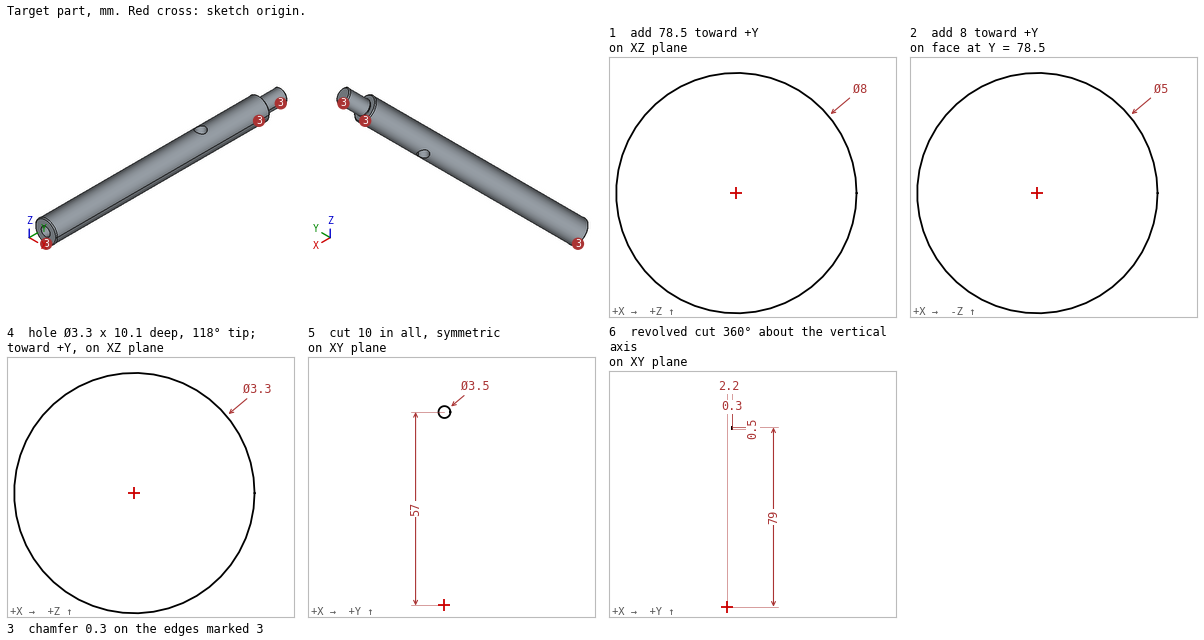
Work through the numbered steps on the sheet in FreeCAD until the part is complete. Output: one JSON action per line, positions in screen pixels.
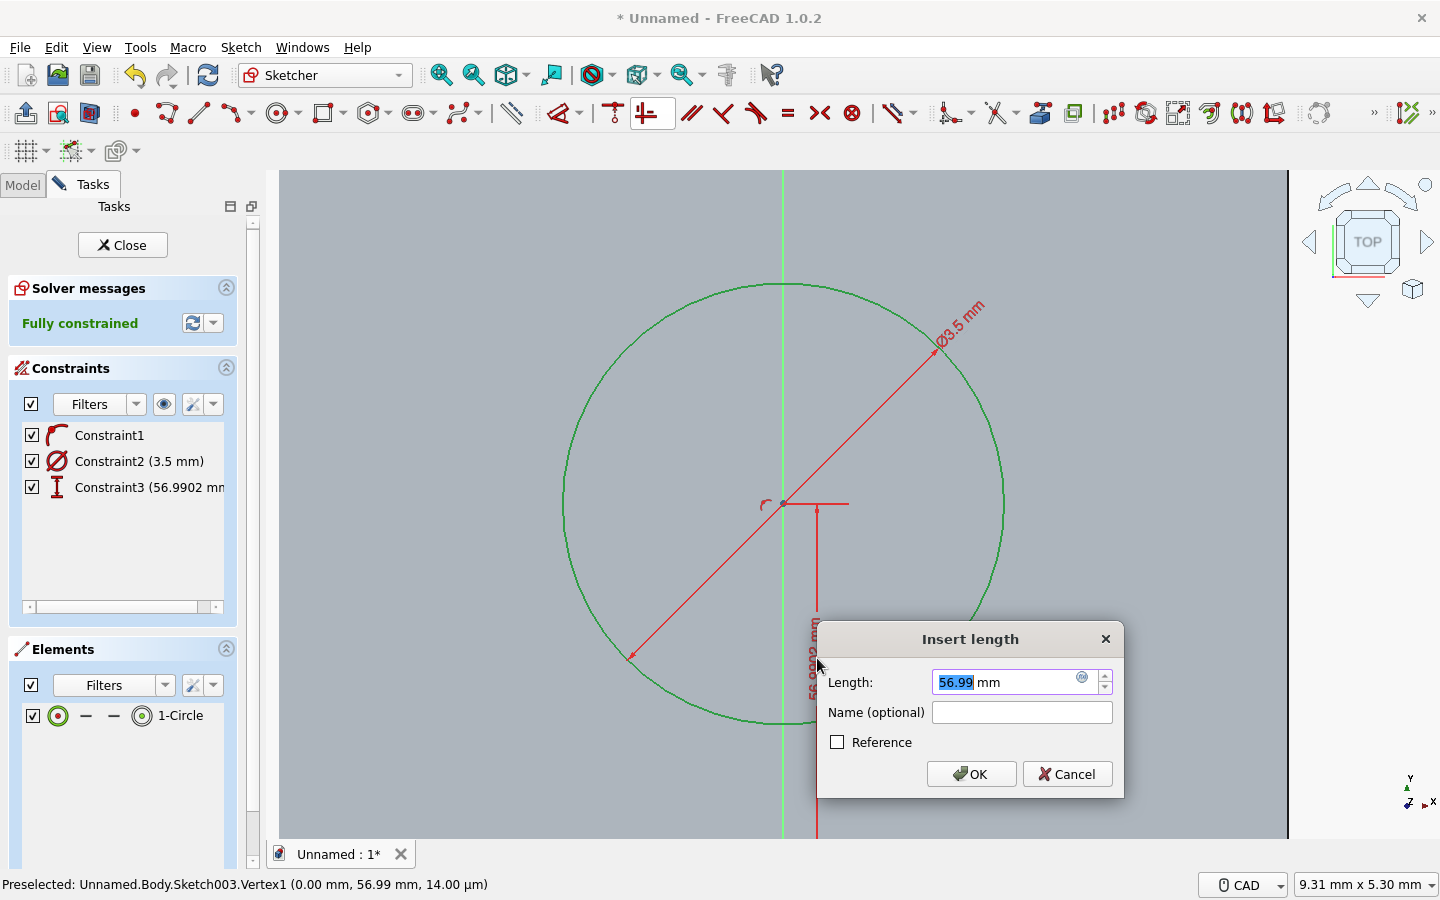
{"action": "type", "text": "57"}
{"action": "key", "text": "Return"}
{"action": "key", "text": "Escape"}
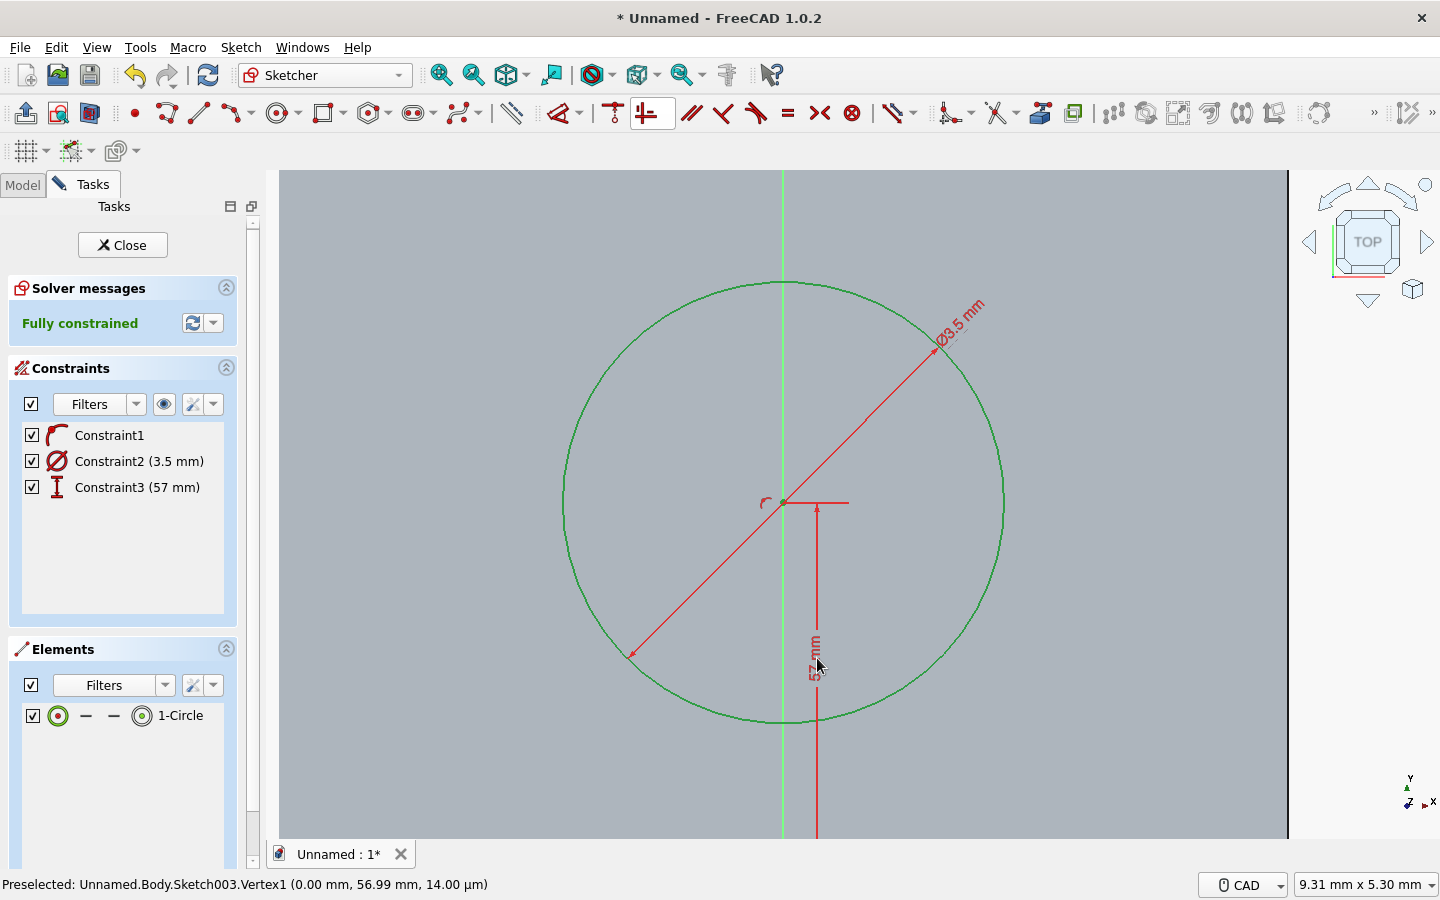
{"action": "left_click", "coordinate": [123, 245]}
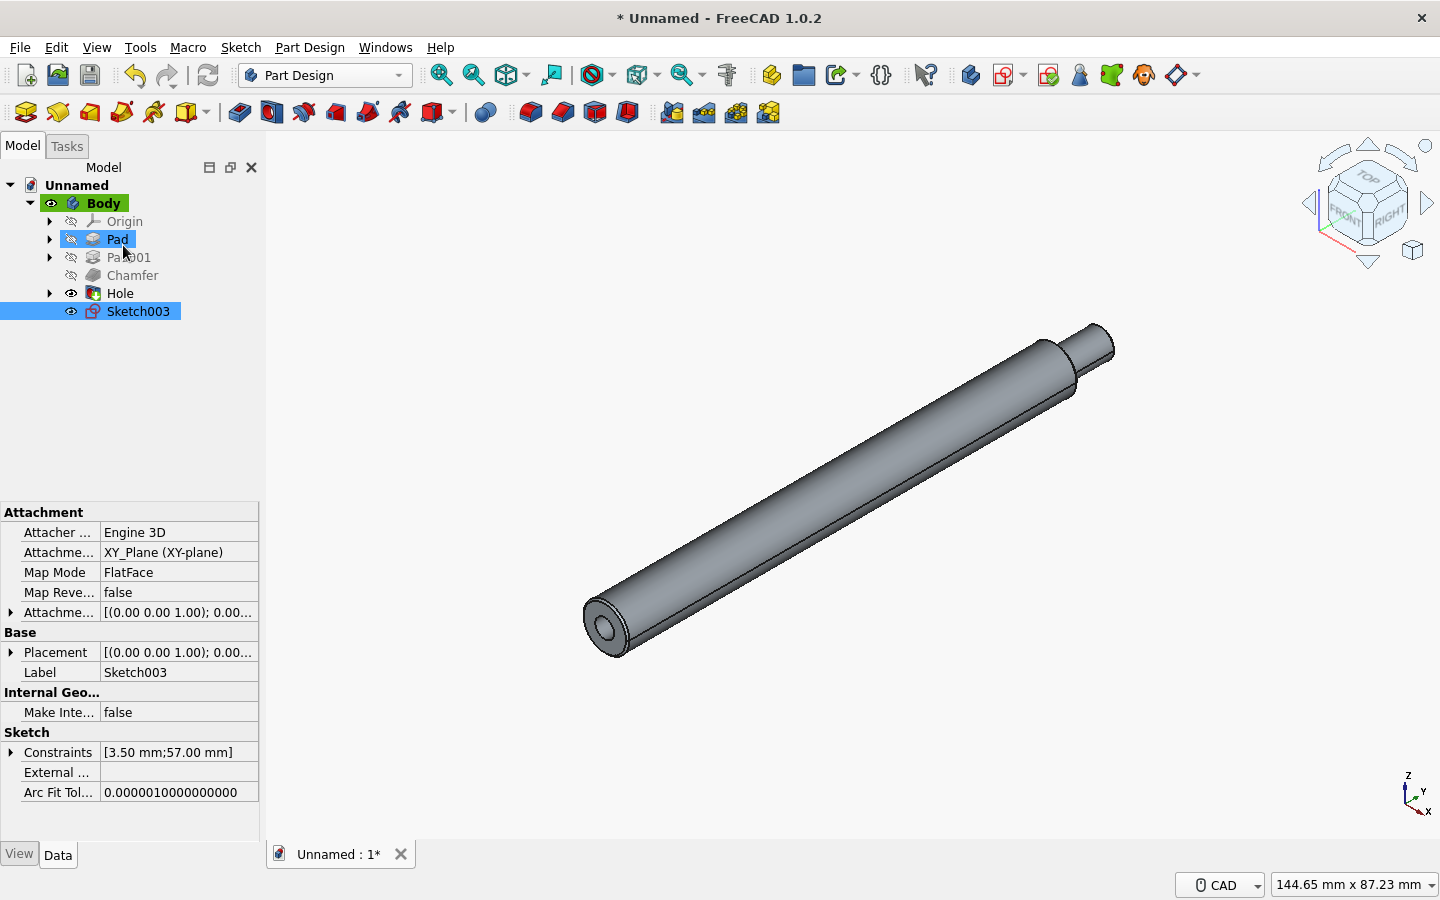
{"action": "left_click", "coordinate": [240, 112]}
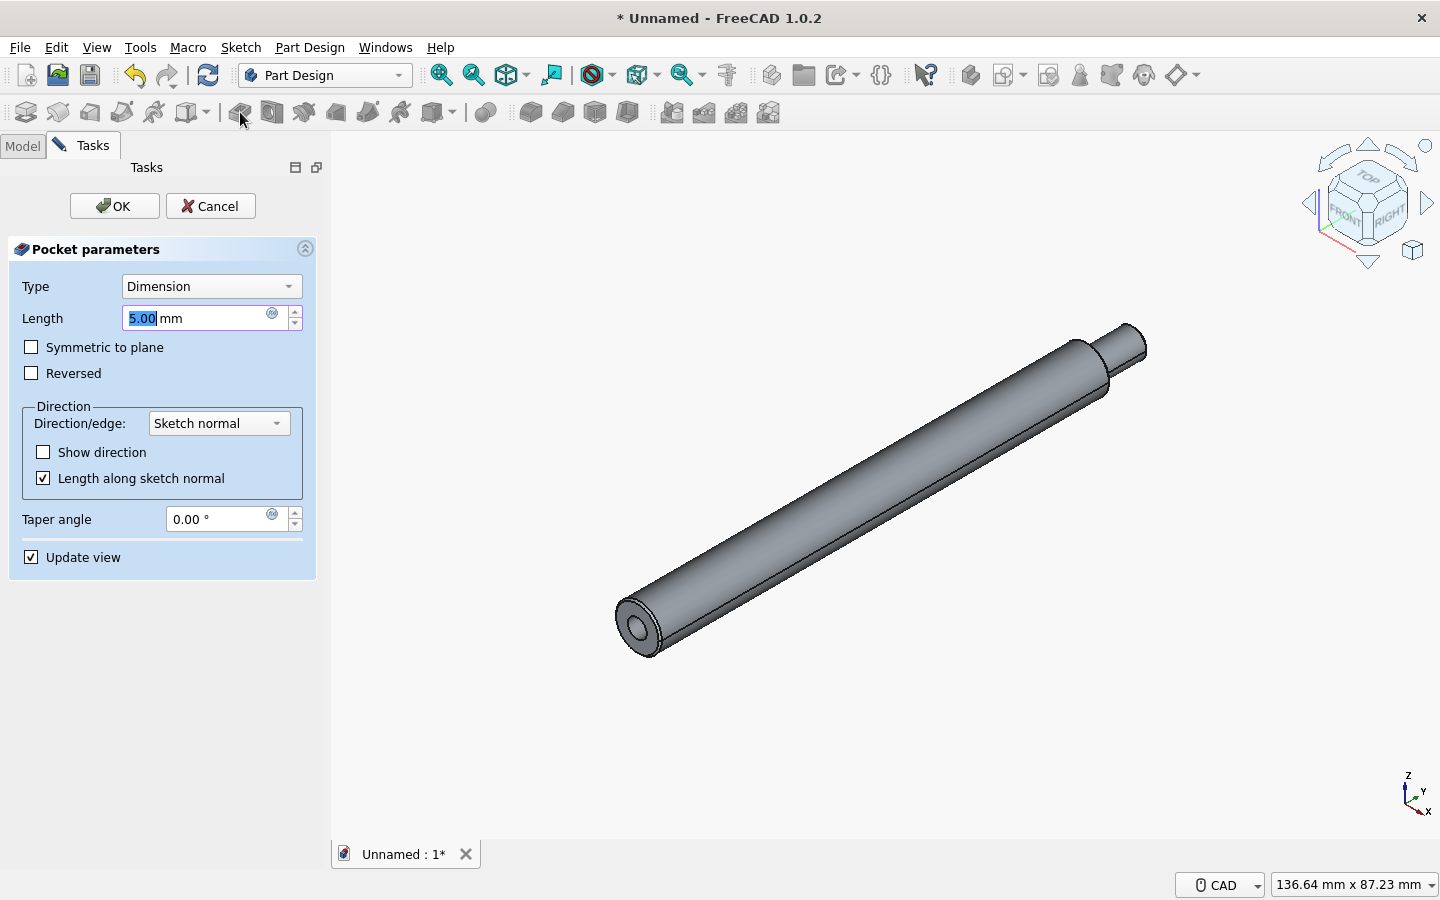
{"action": "type", "text": "10"}
{"action": "key", "text": "Tab"}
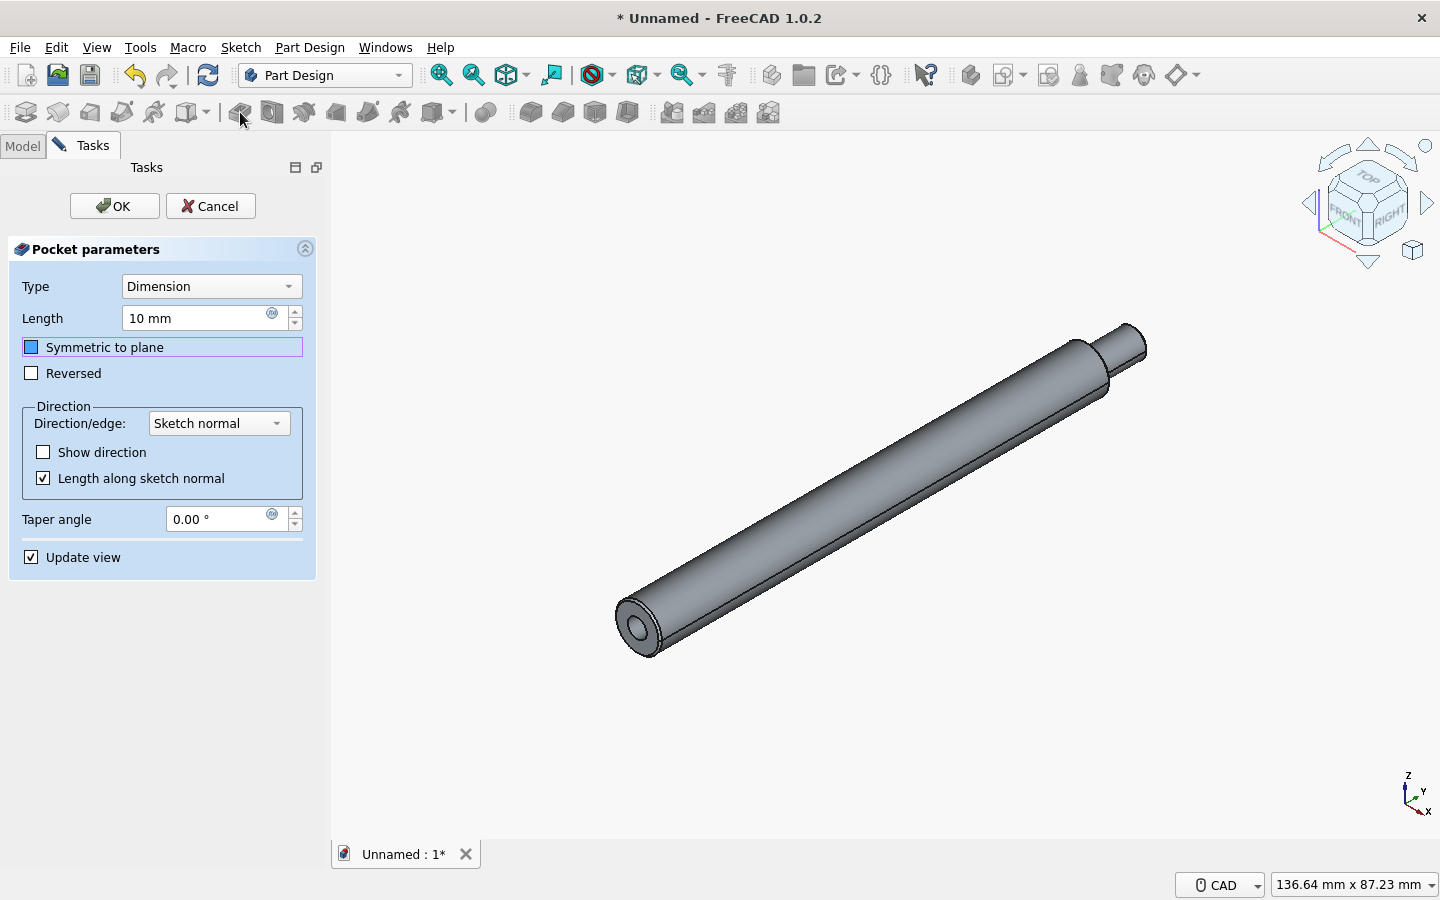
{"action": "left_click", "coordinate": [30, 347]}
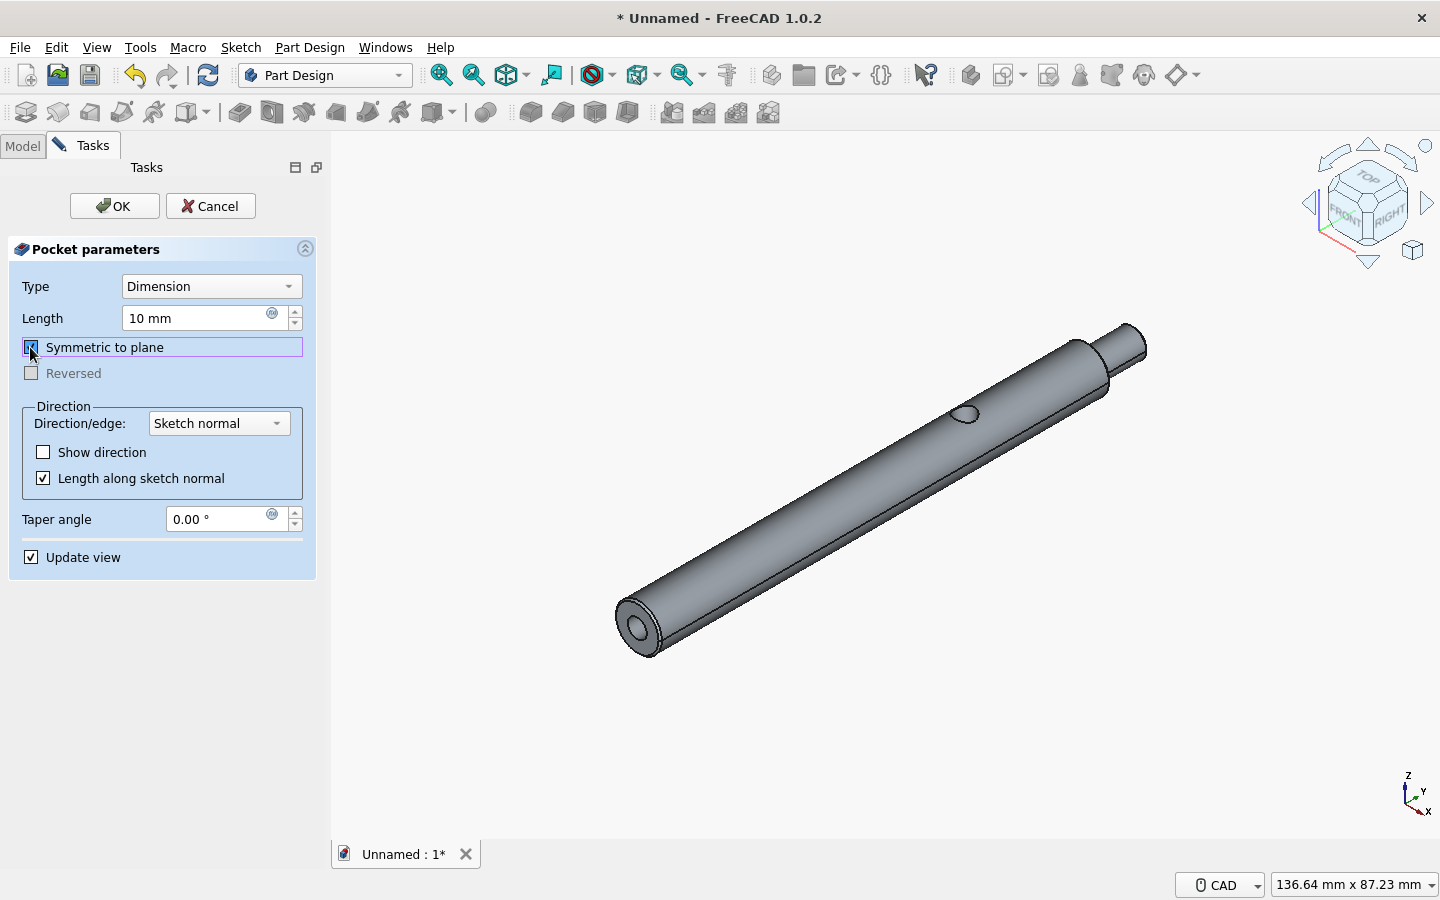
{"action": "left_click", "coordinate": [115, 206]}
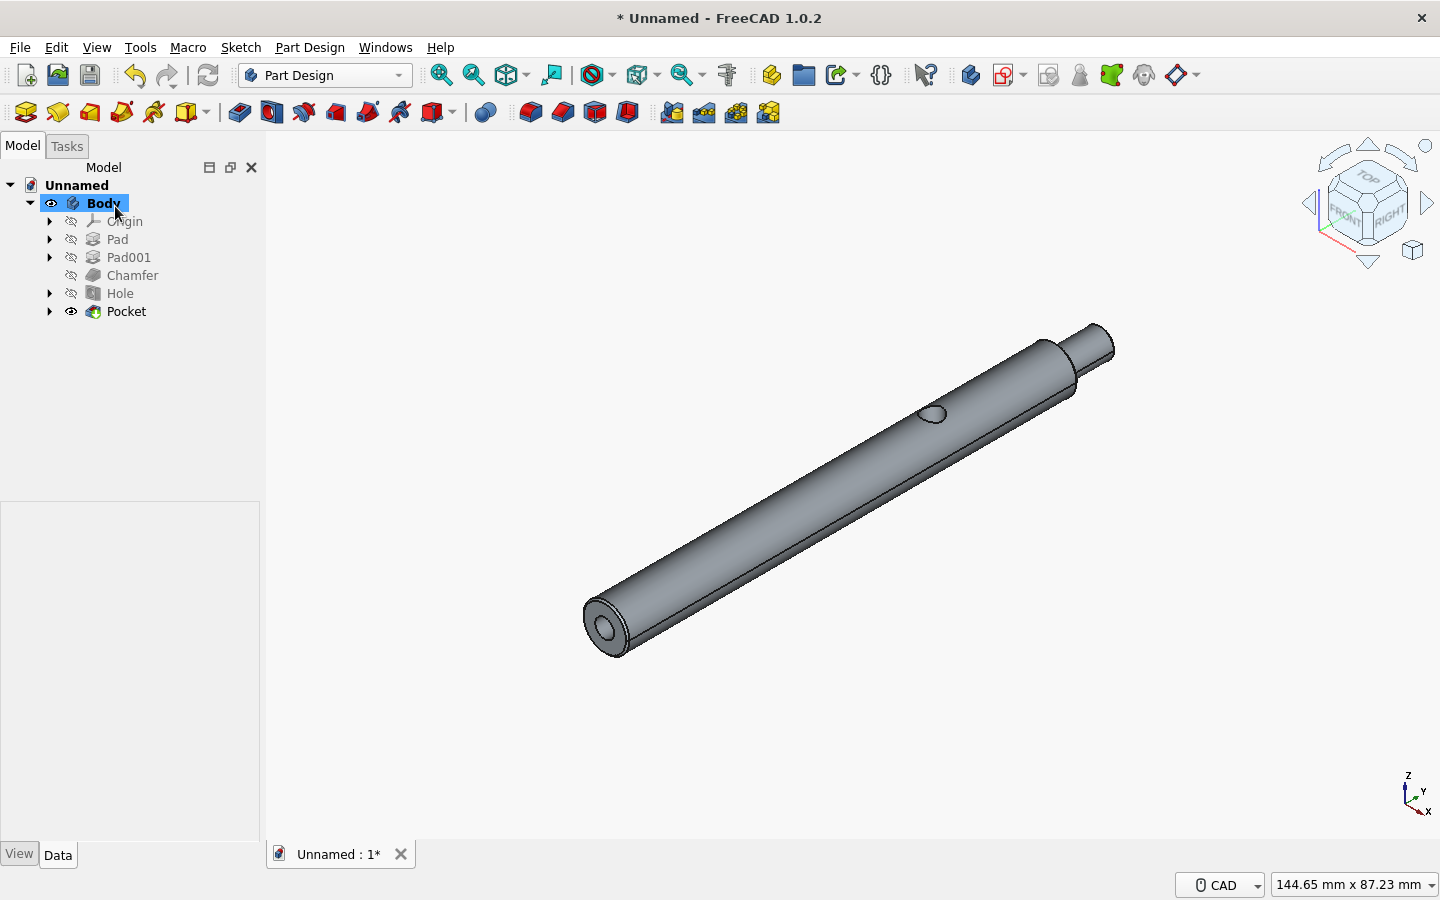
{"action": "left_click", "coordinate": [1004, 76]}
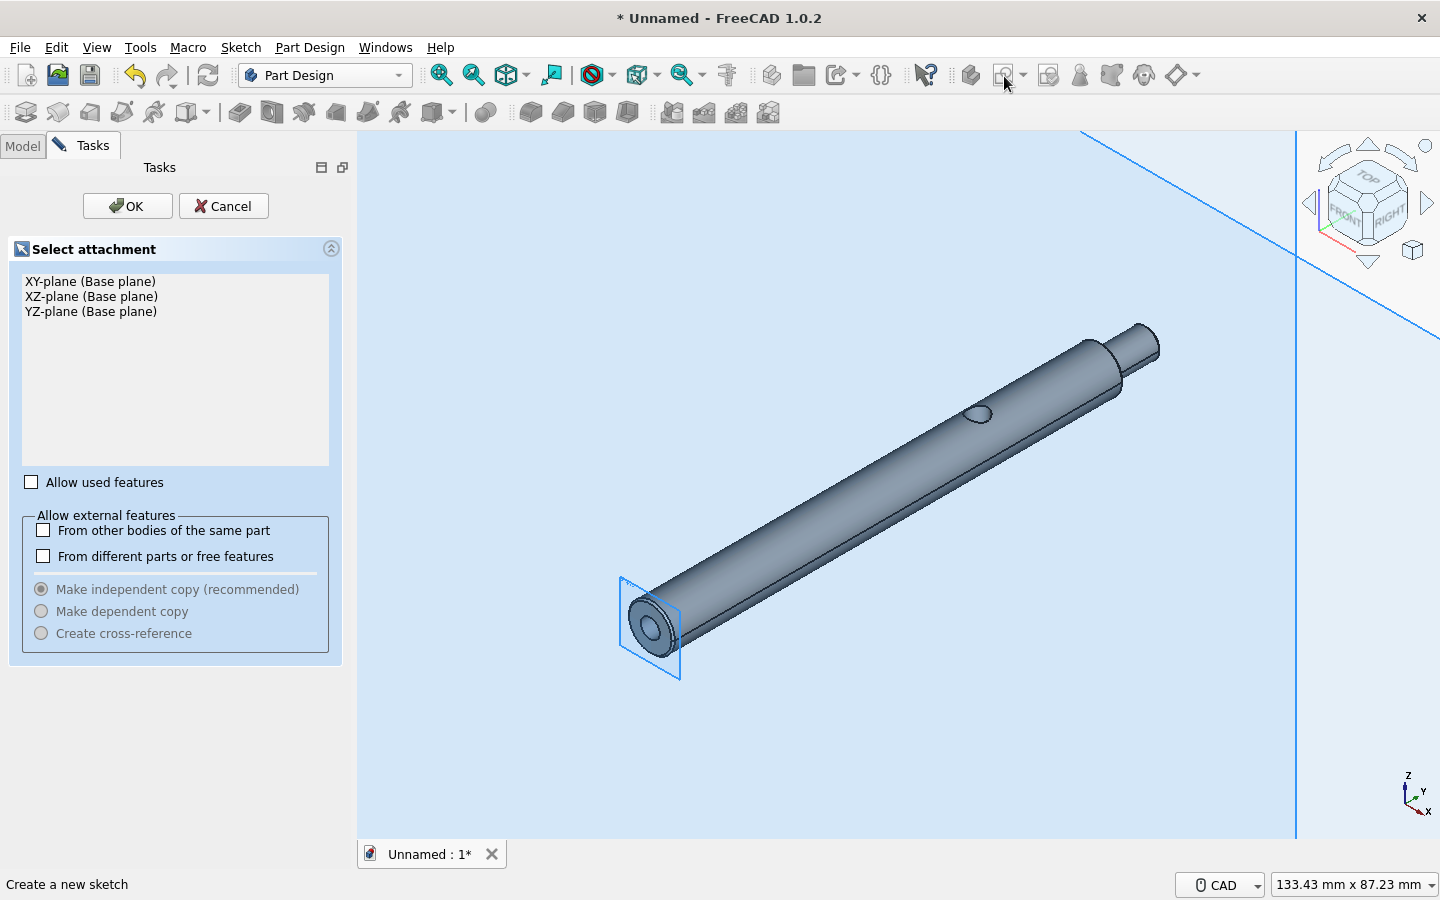
{"action": "left_click", "coordinate": [82, 282]}